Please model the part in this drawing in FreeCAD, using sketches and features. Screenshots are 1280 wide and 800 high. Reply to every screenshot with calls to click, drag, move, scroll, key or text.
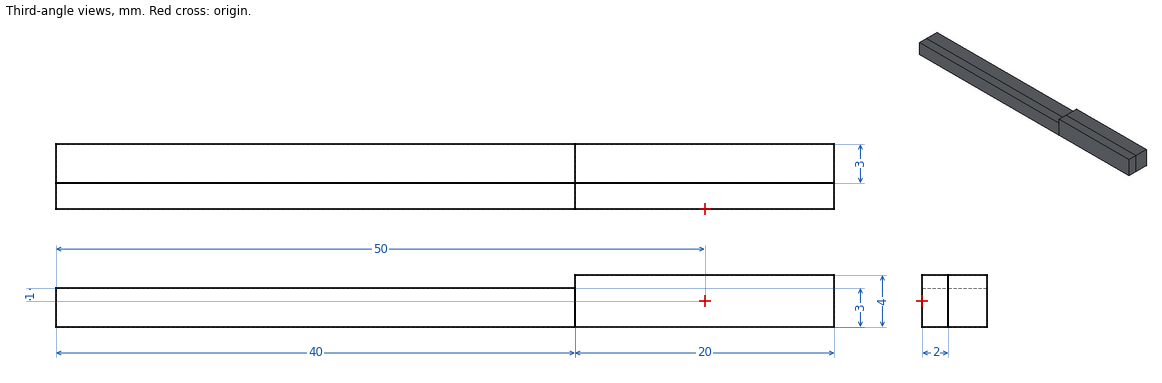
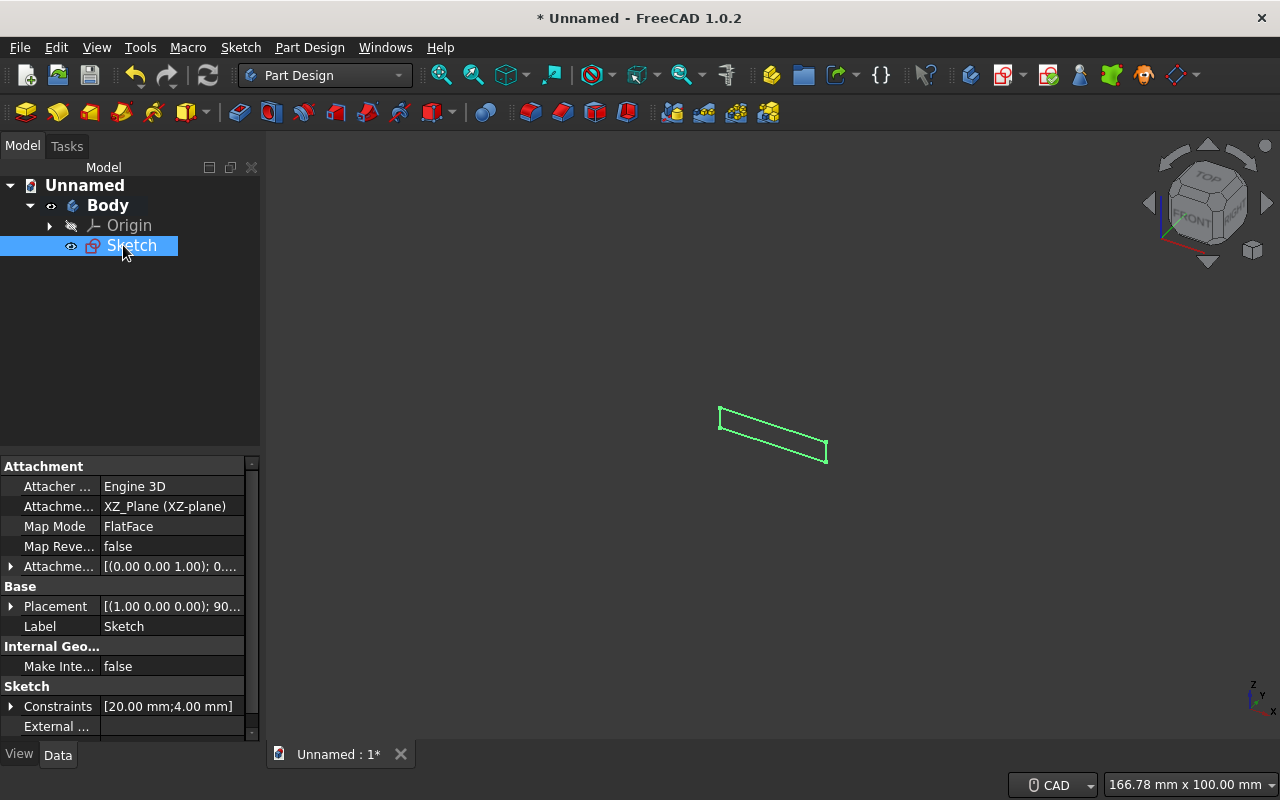
click(26, 112)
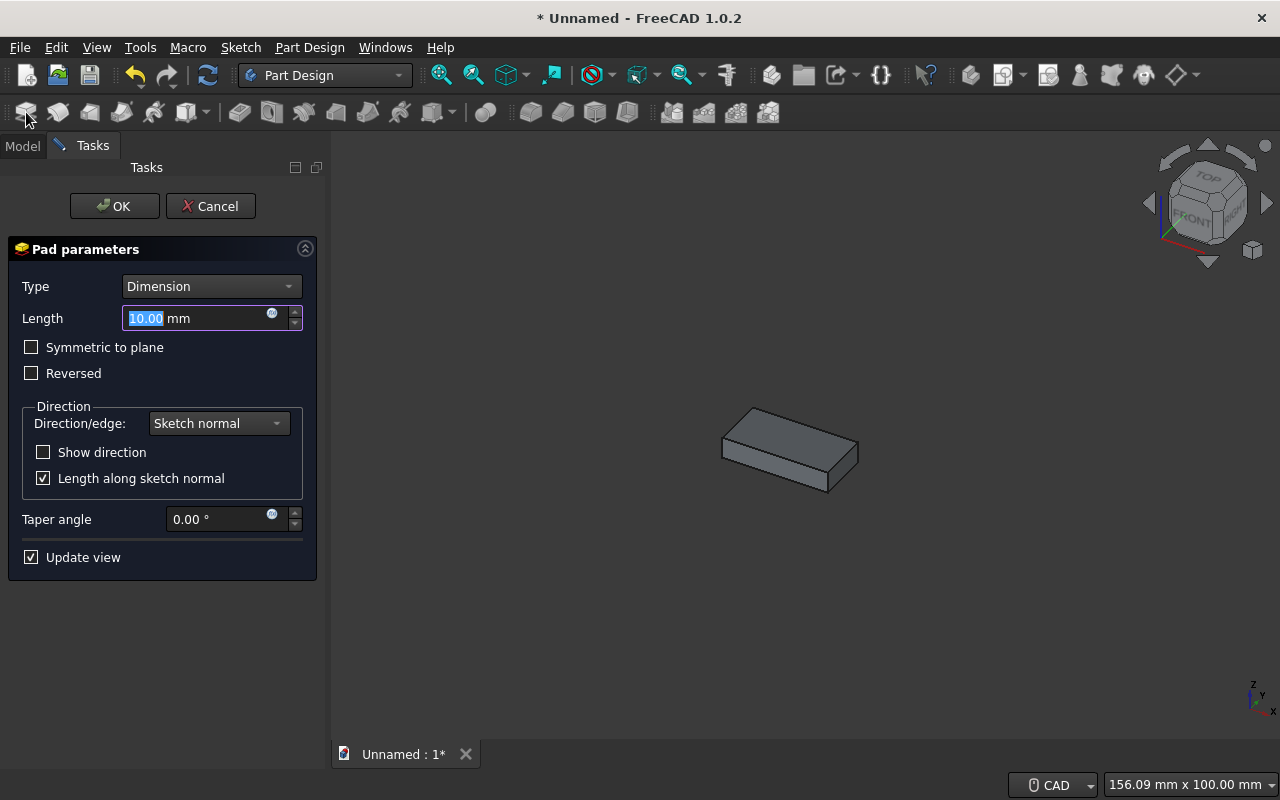
text(2)
key(Tab)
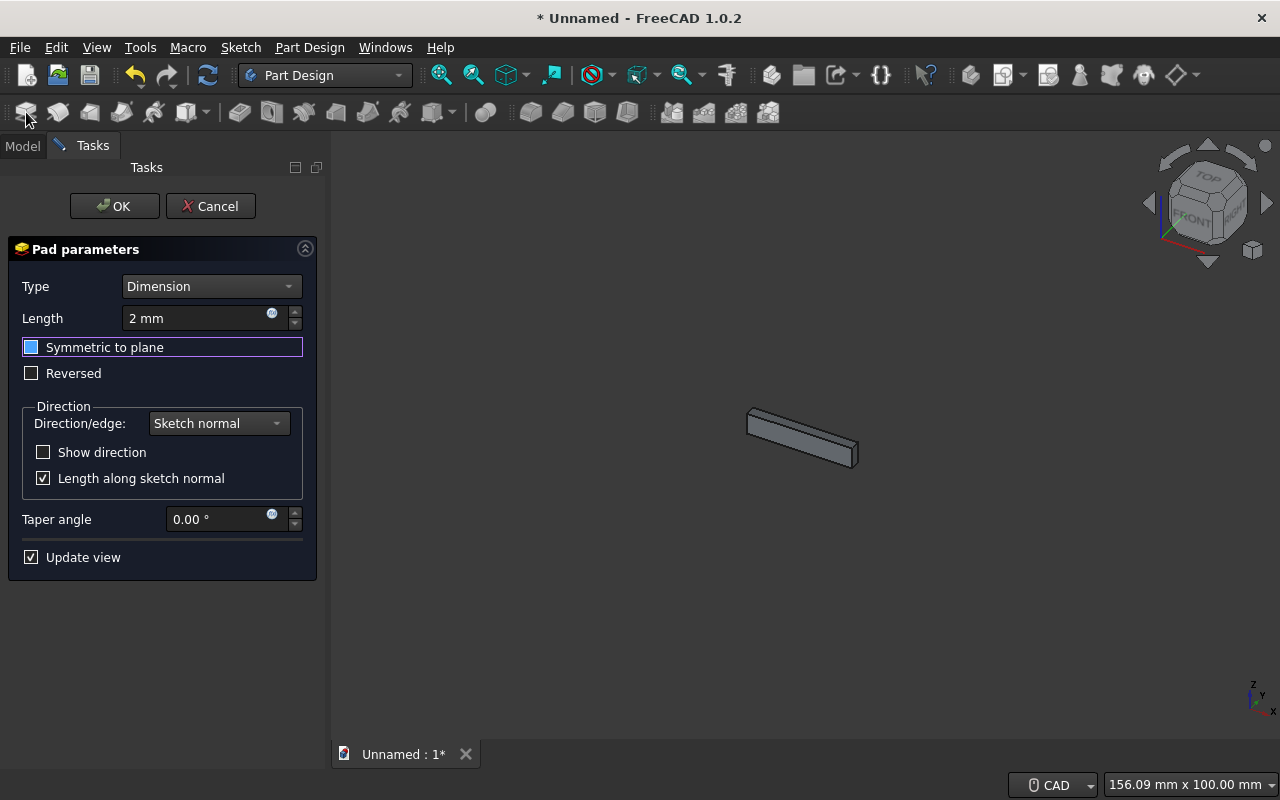
click(30, 373)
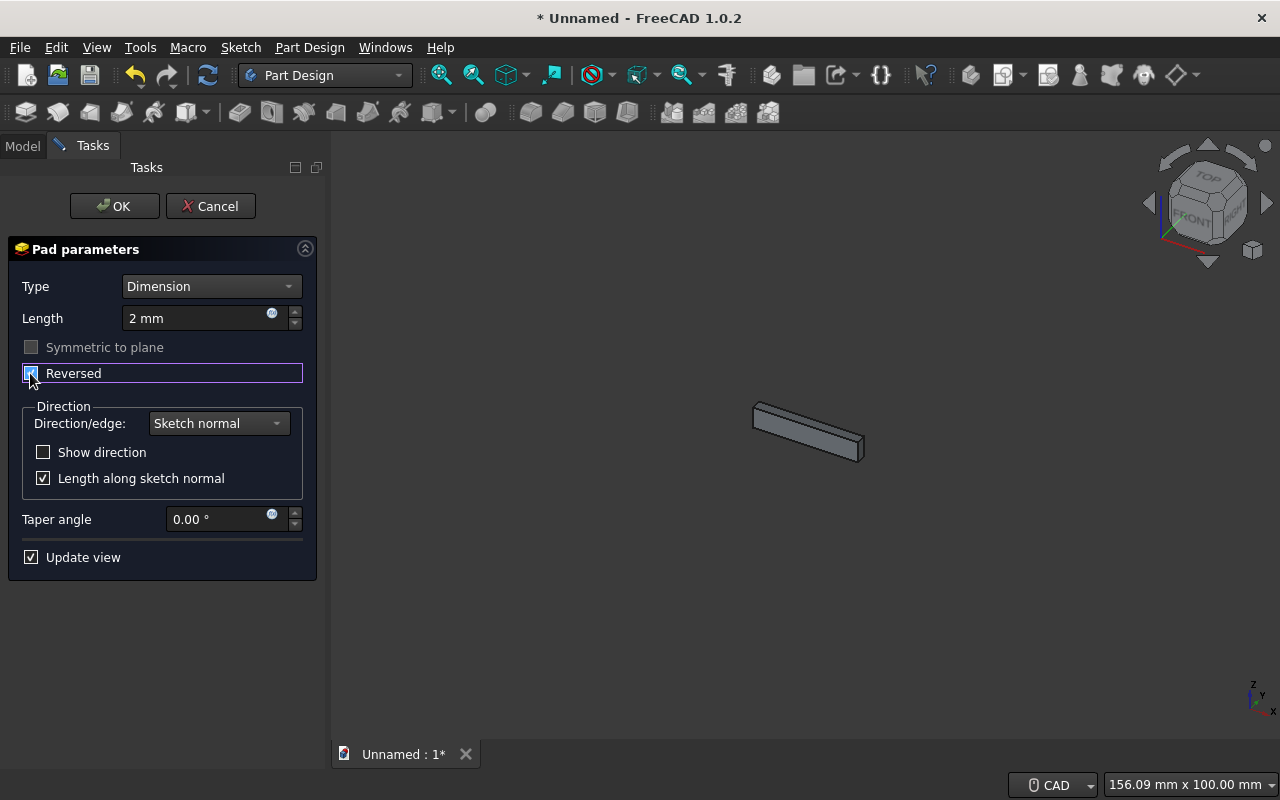
click(115, 206)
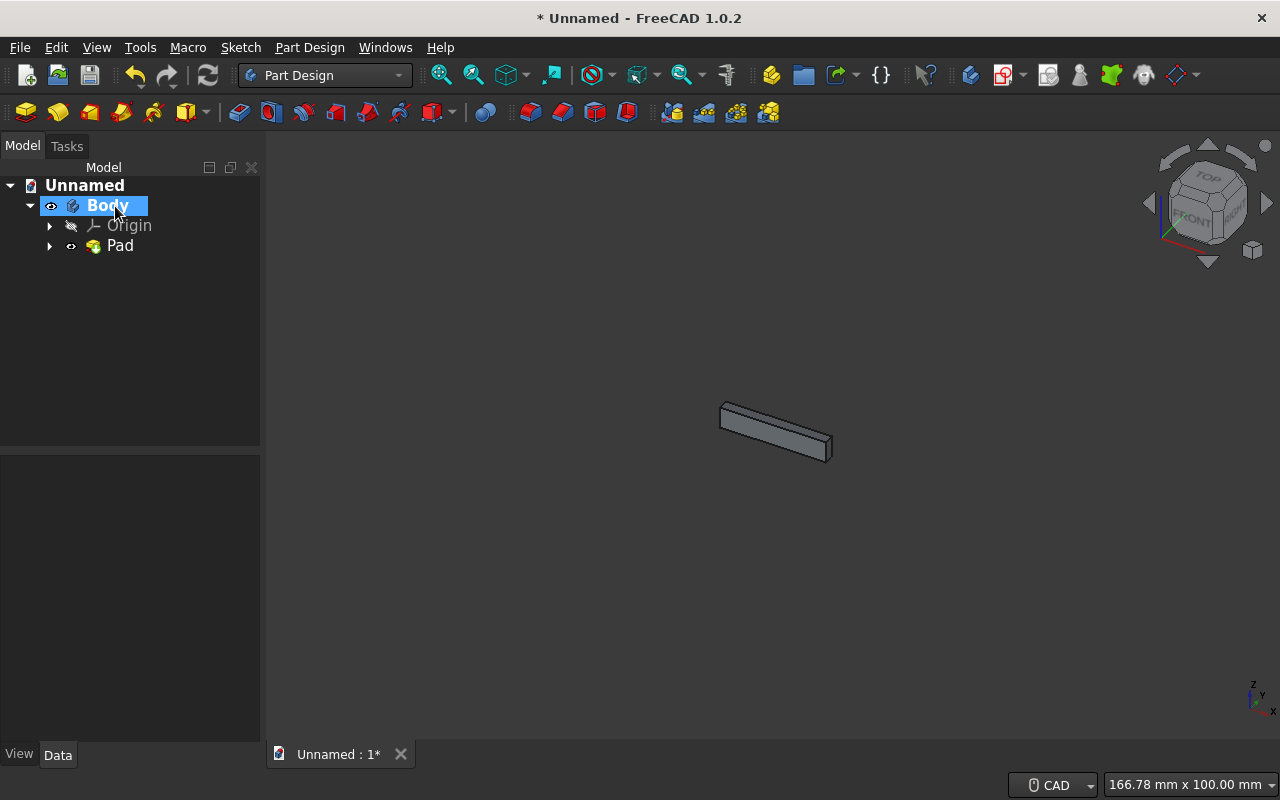
click(442, 76)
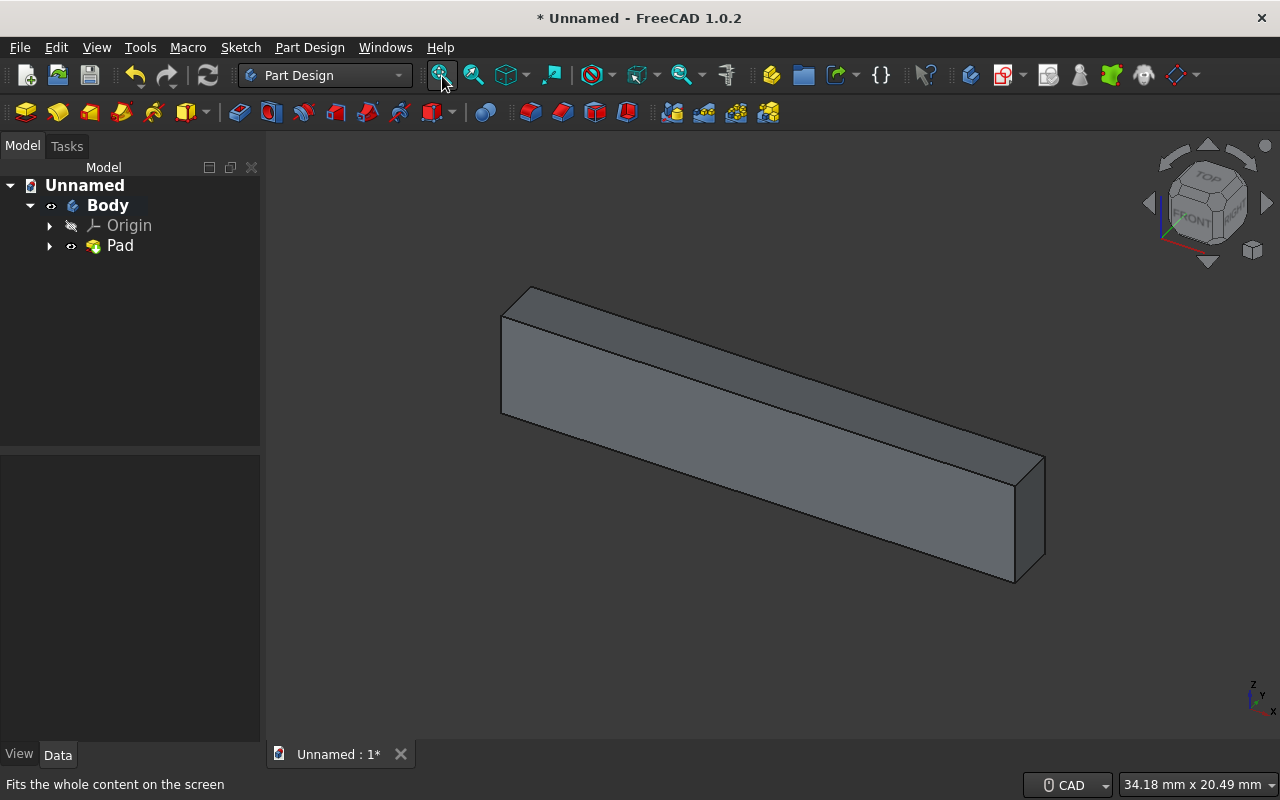
click(972, 76)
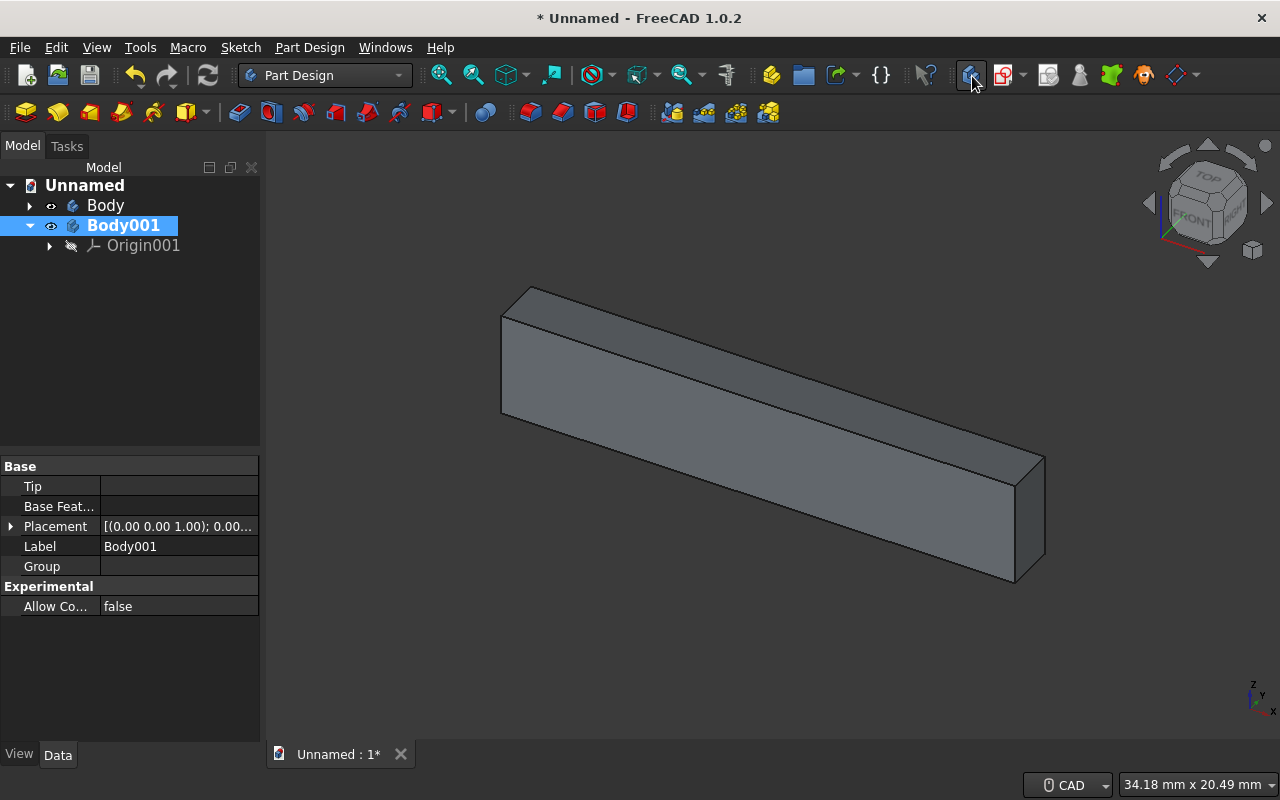
click(50, 246)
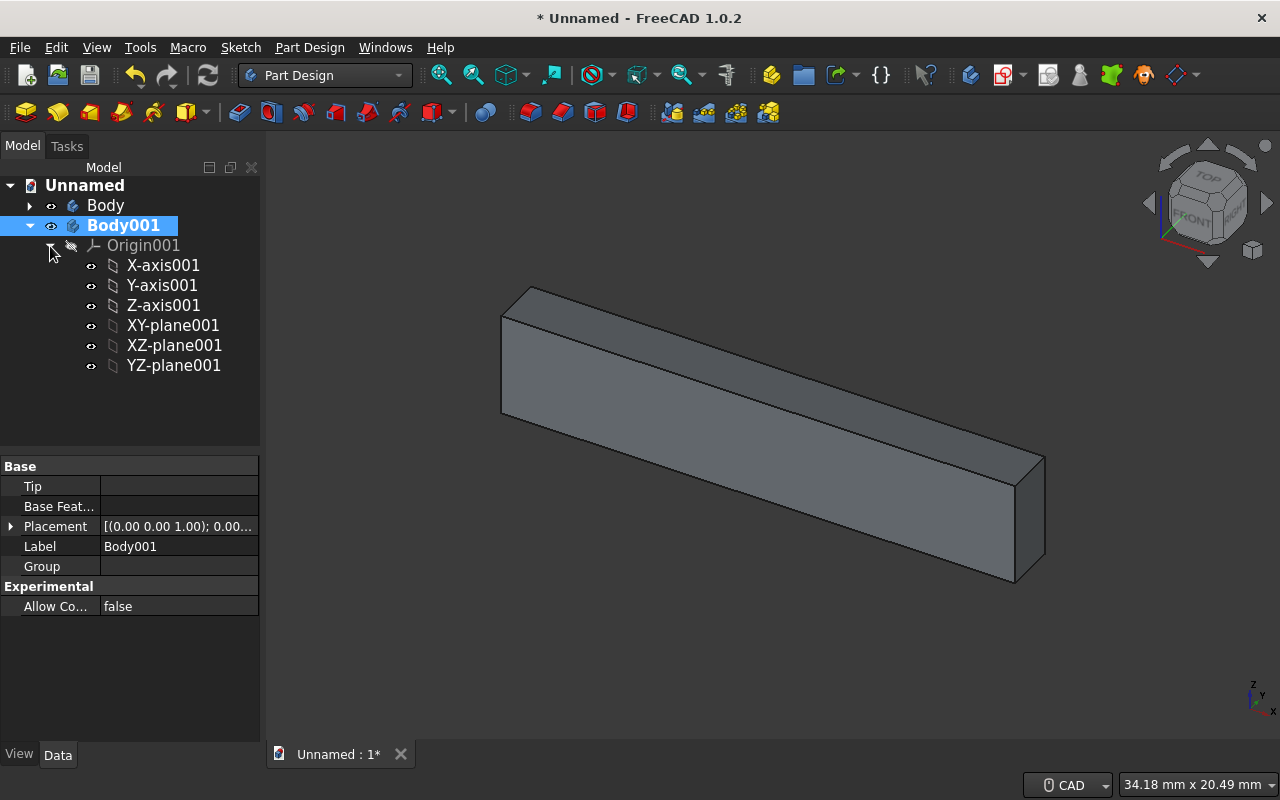
click(136, 346)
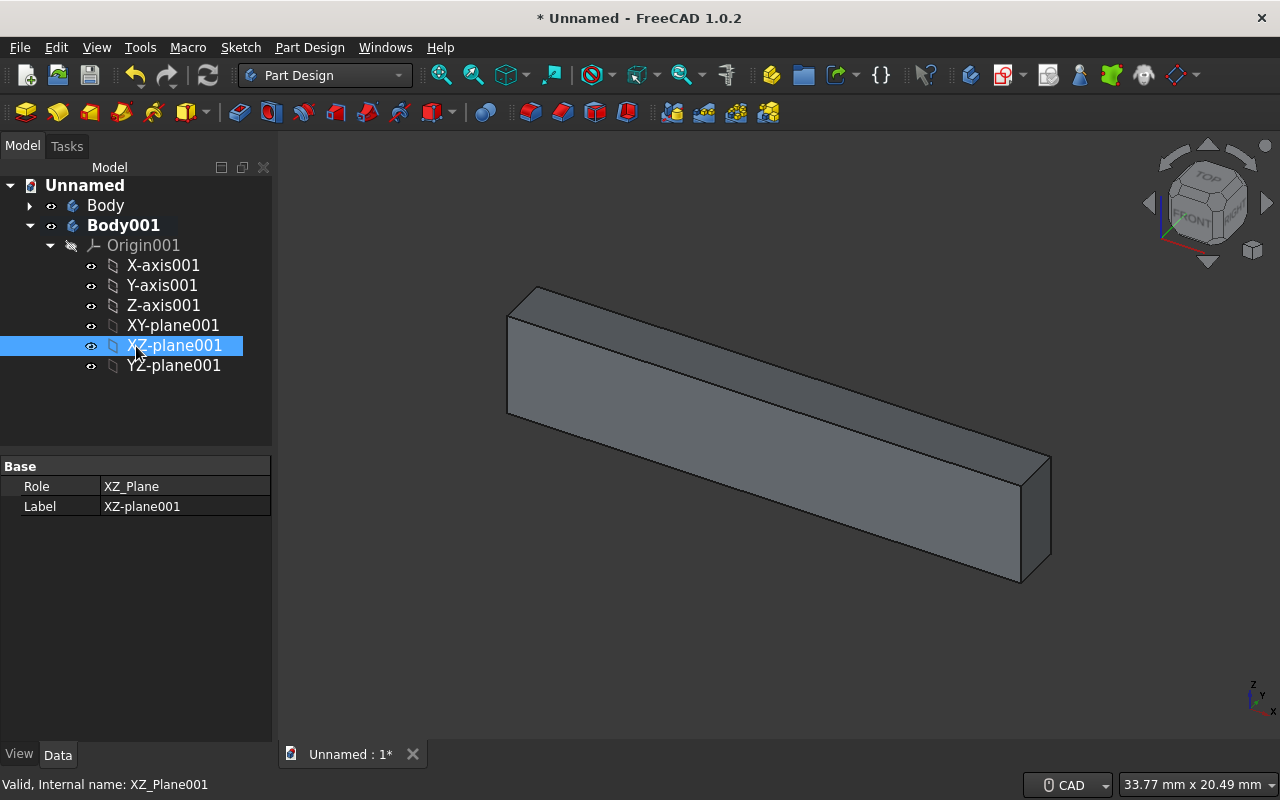
click(1176, 76)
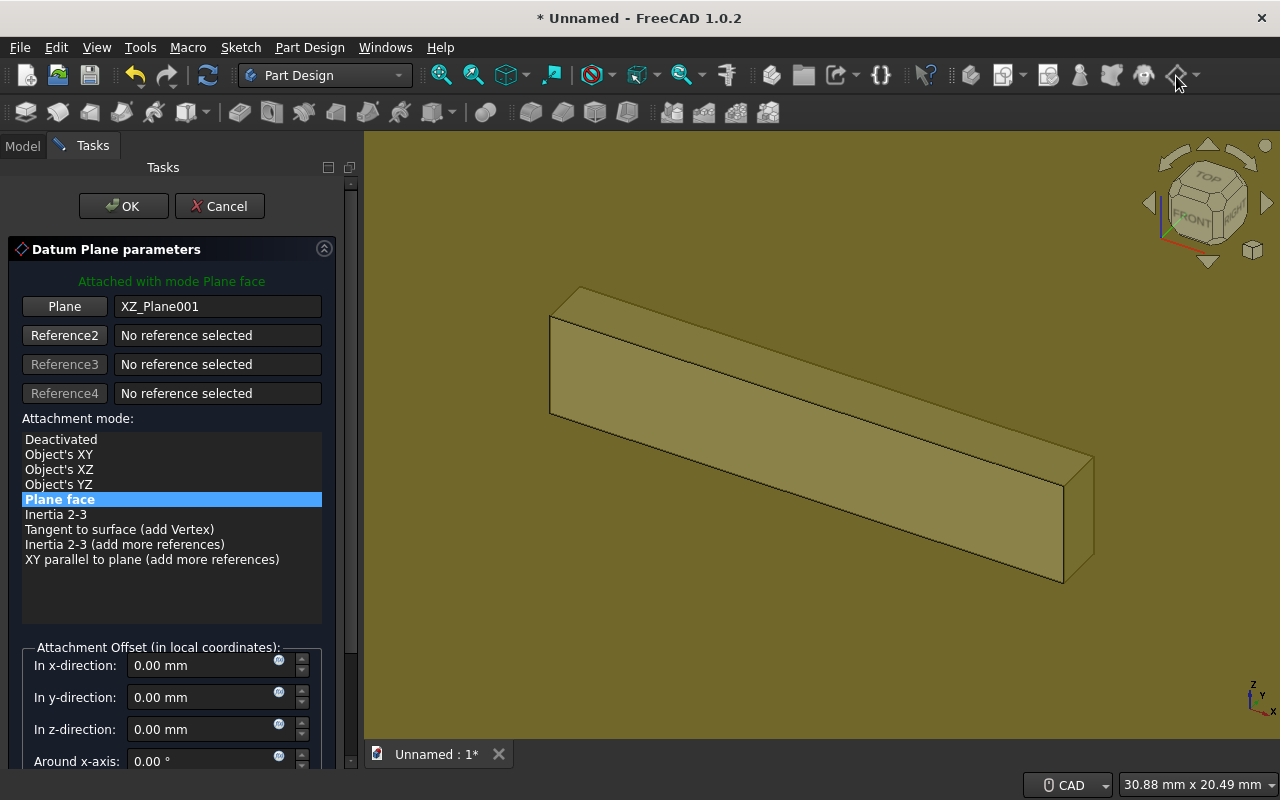
triple_click(210, 729)